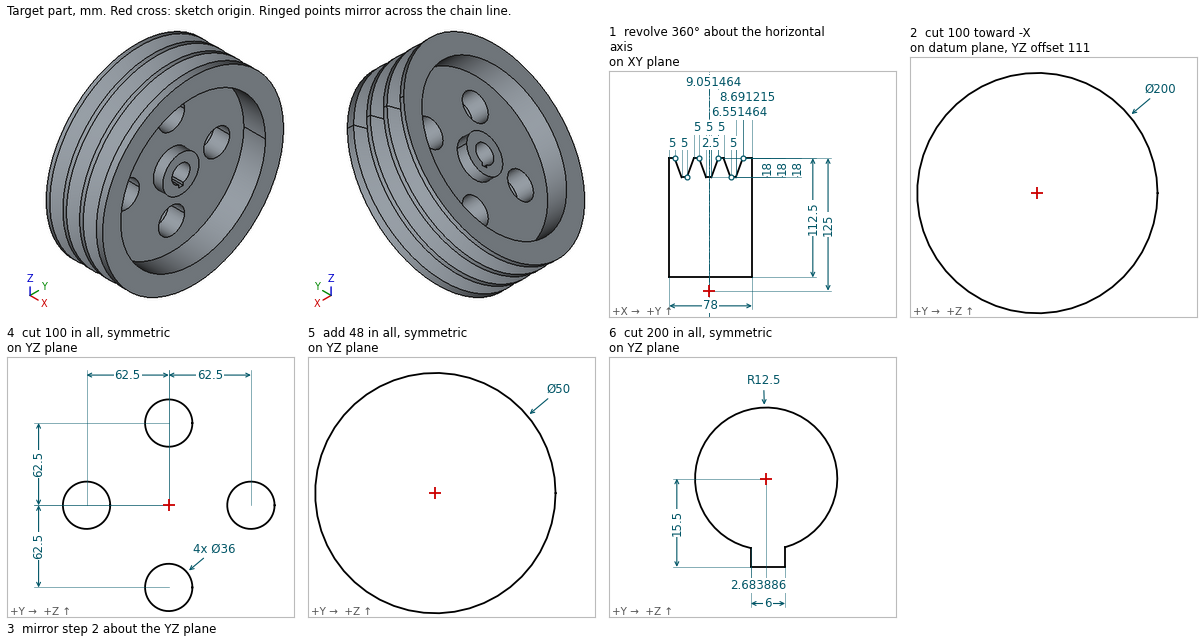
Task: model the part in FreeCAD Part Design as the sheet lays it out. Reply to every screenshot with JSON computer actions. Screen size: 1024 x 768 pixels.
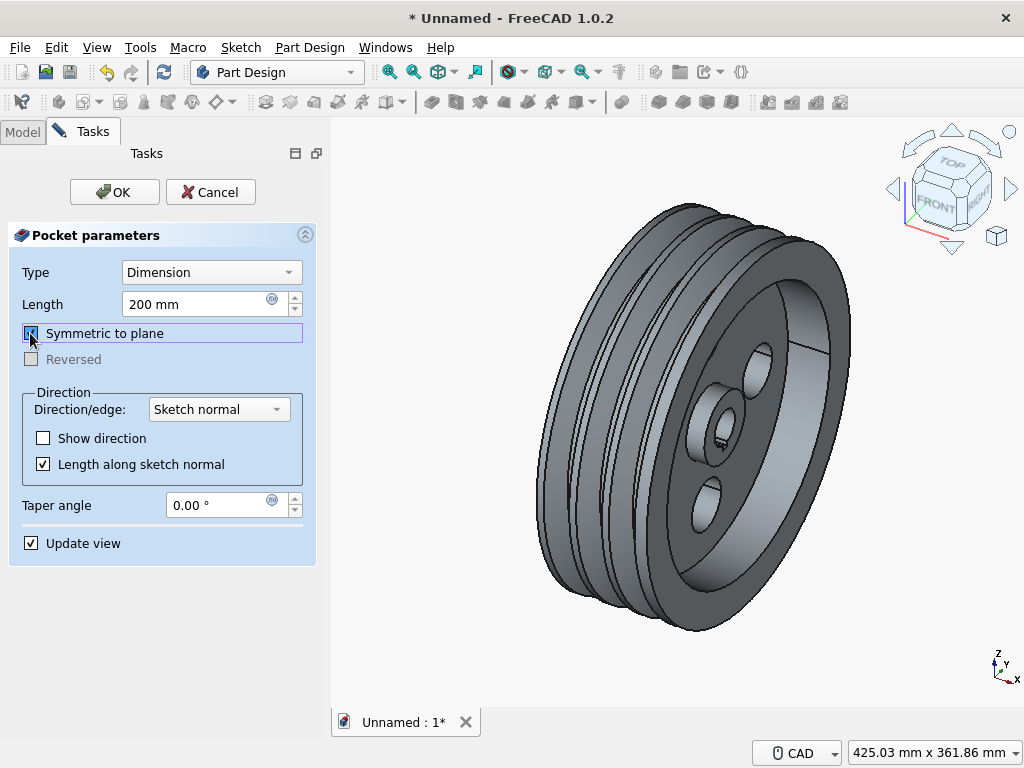
{"action": "left_click", "coordinate": [115, 192]}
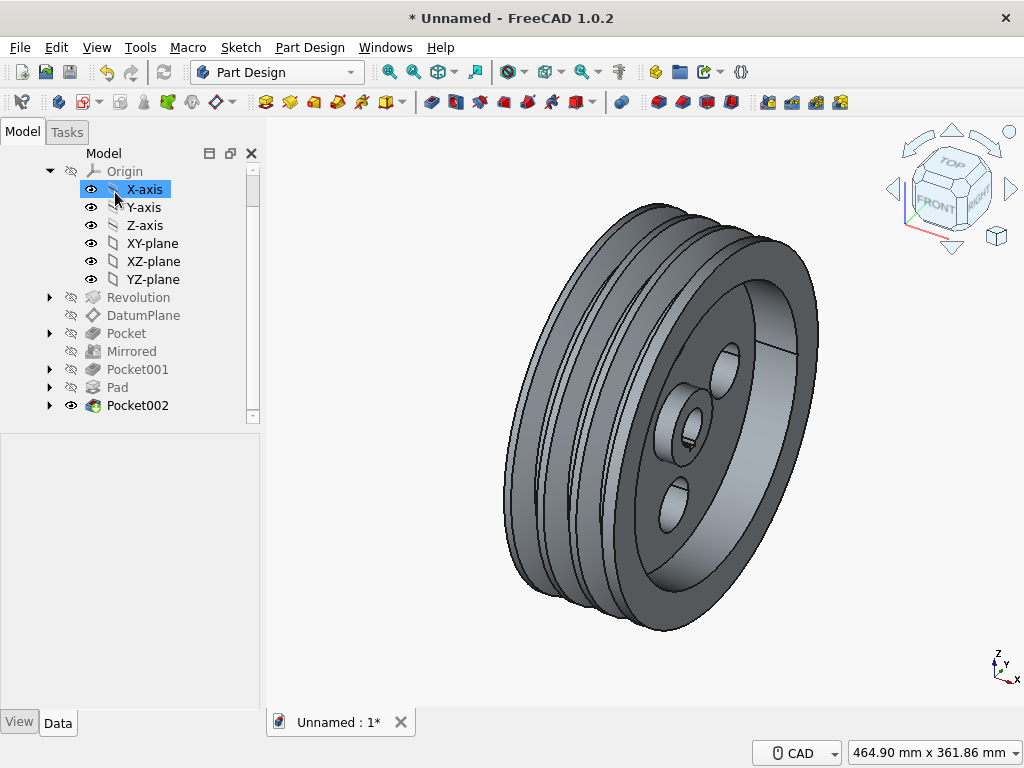
{"action": "key", "text": "0"}